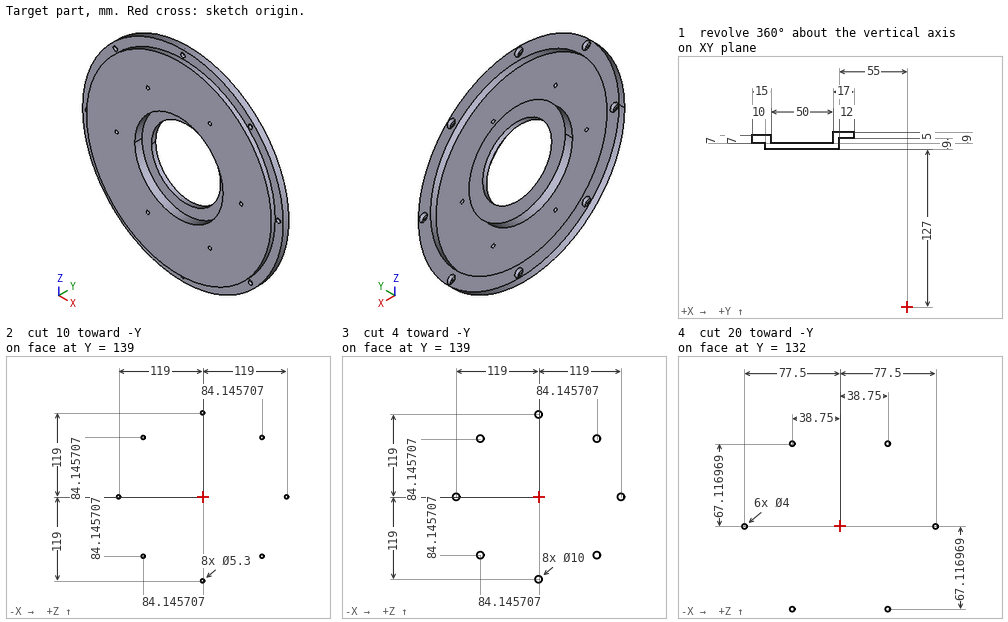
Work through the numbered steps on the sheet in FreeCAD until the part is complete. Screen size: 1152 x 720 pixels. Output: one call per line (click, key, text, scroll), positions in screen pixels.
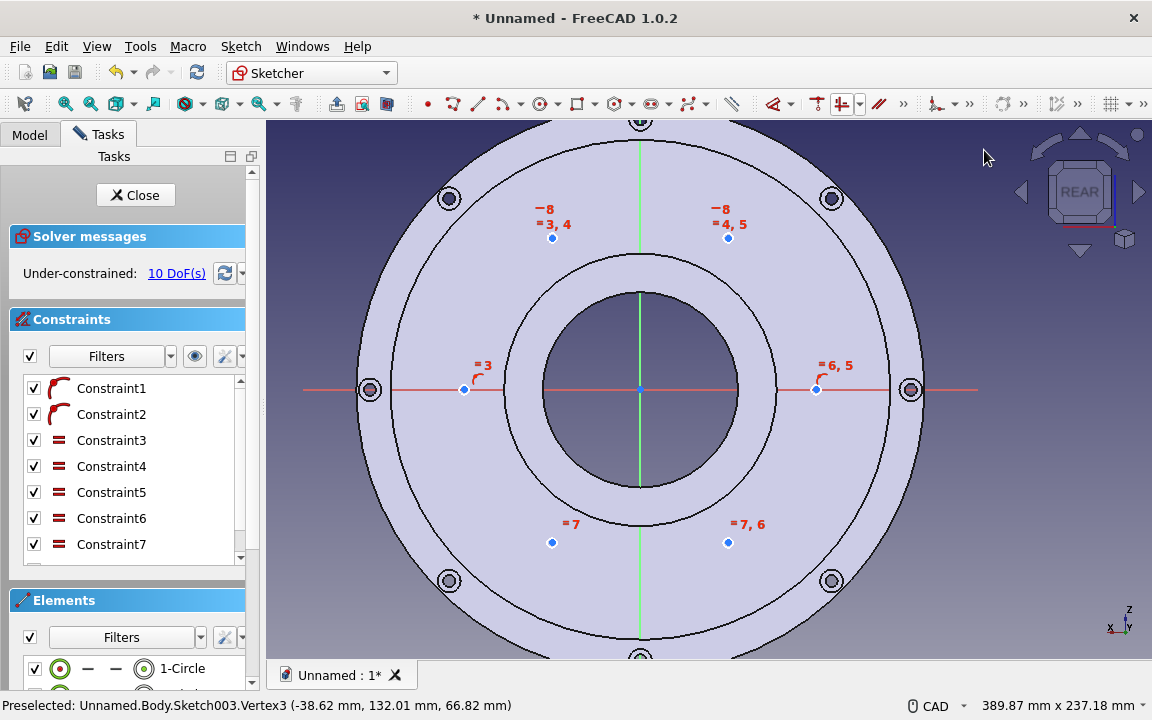
click(728, 238)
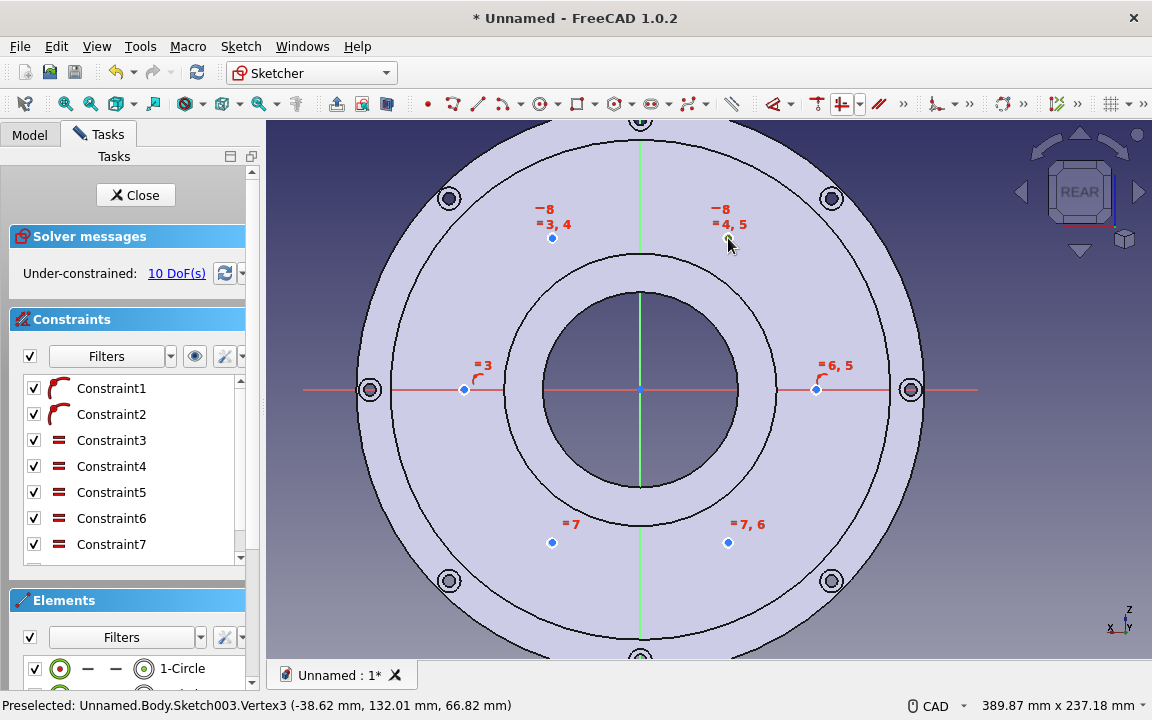
click(728, 543)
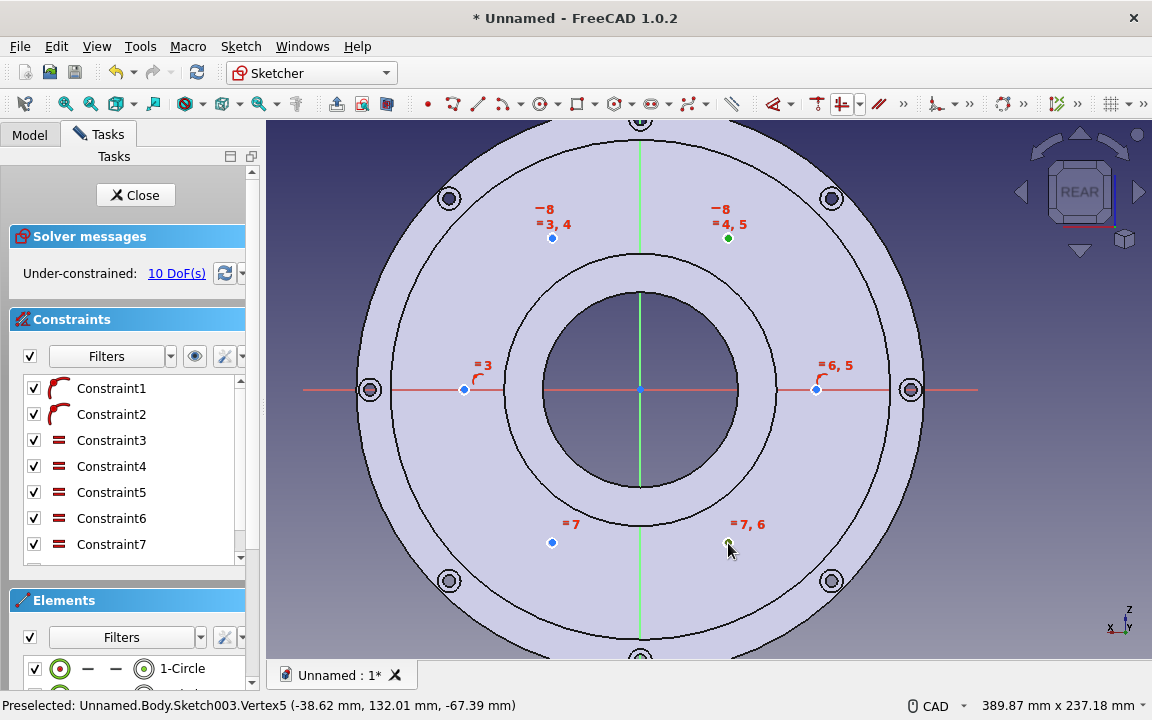
key(v)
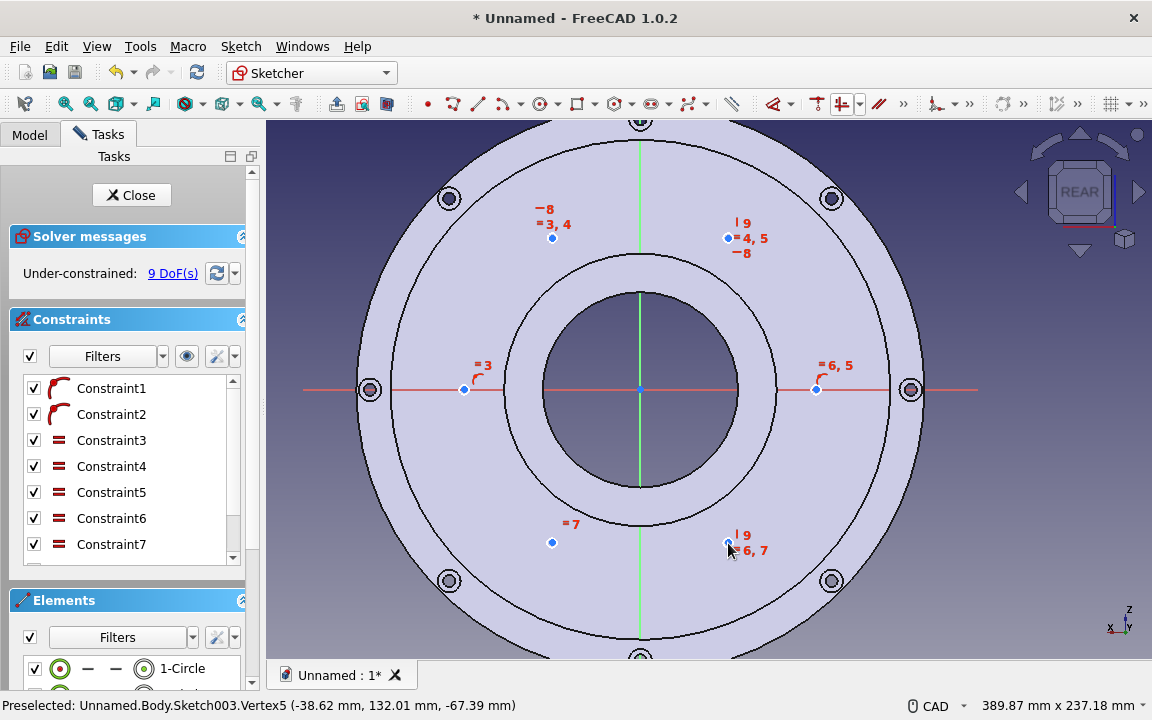
click(552, 238)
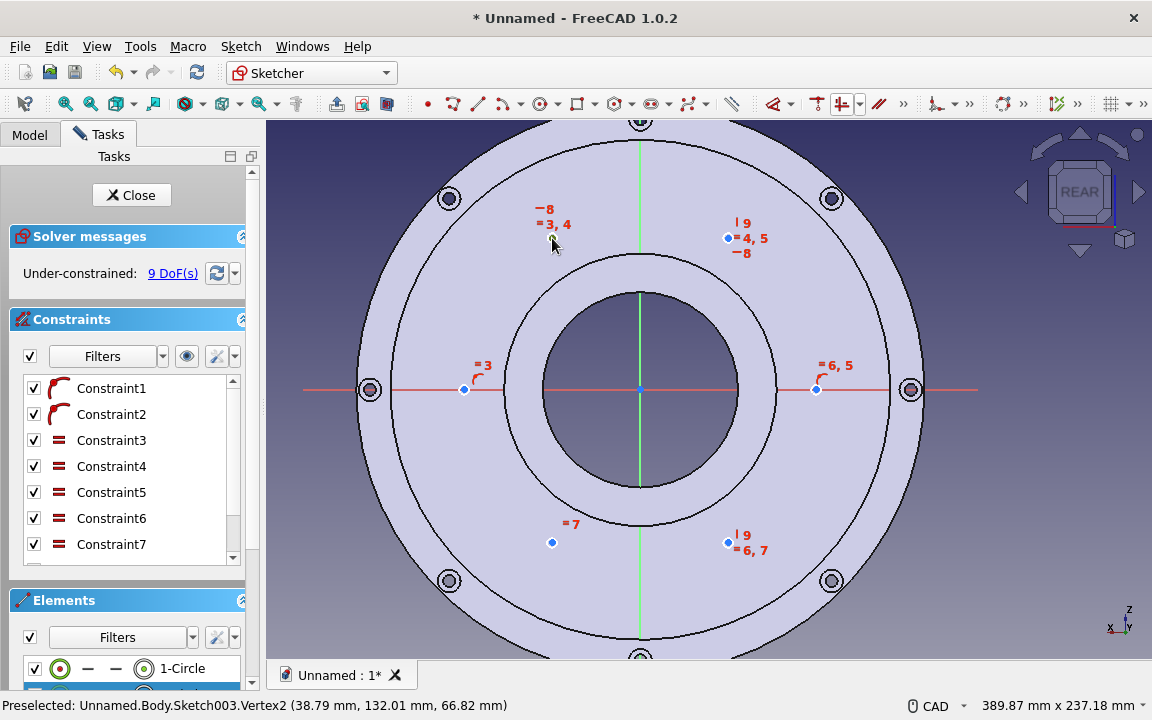
click(552, 543)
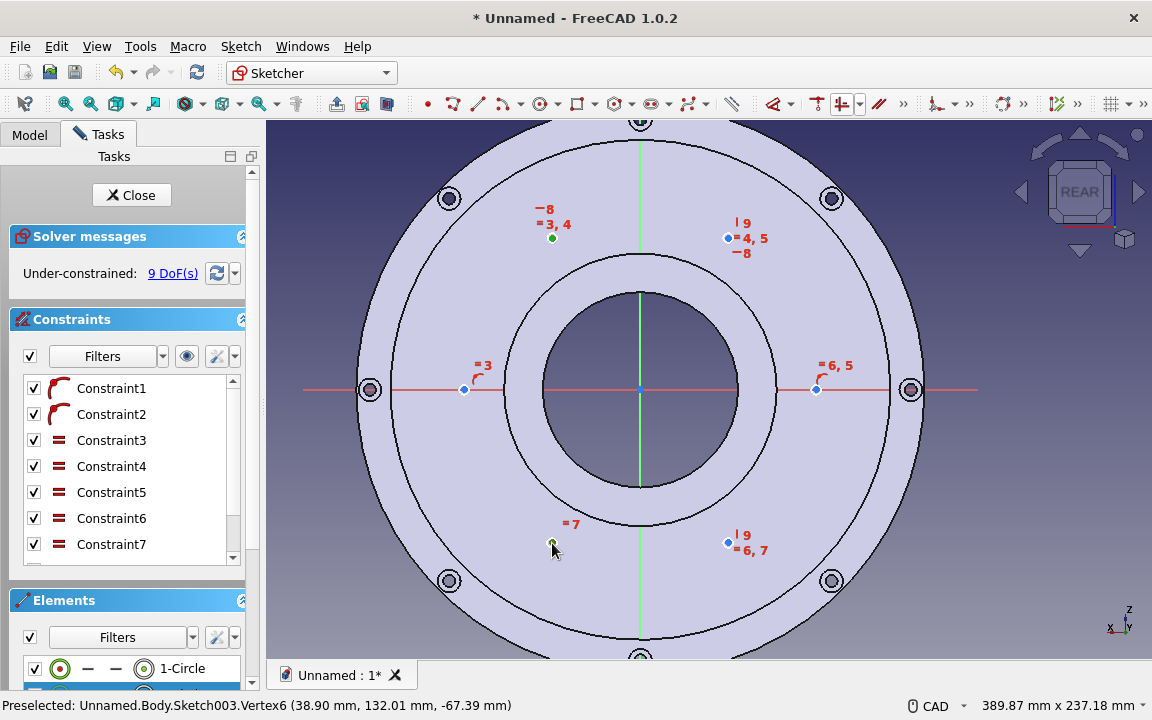
click(860, 104)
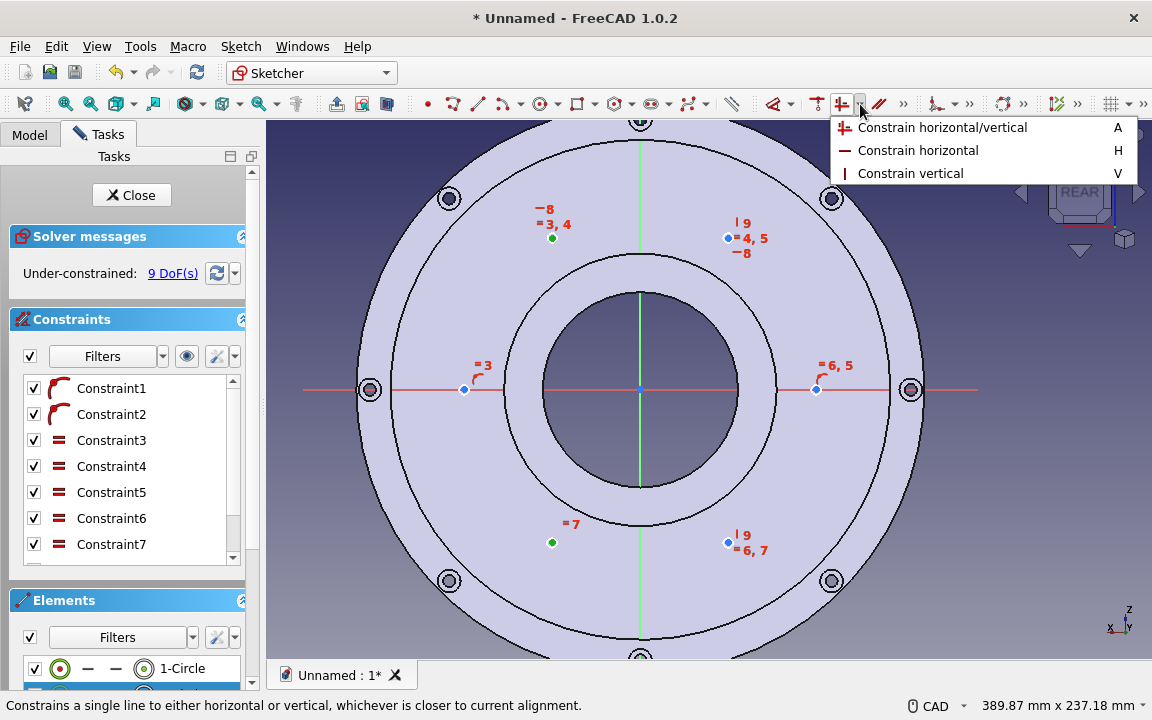
click(984, 174)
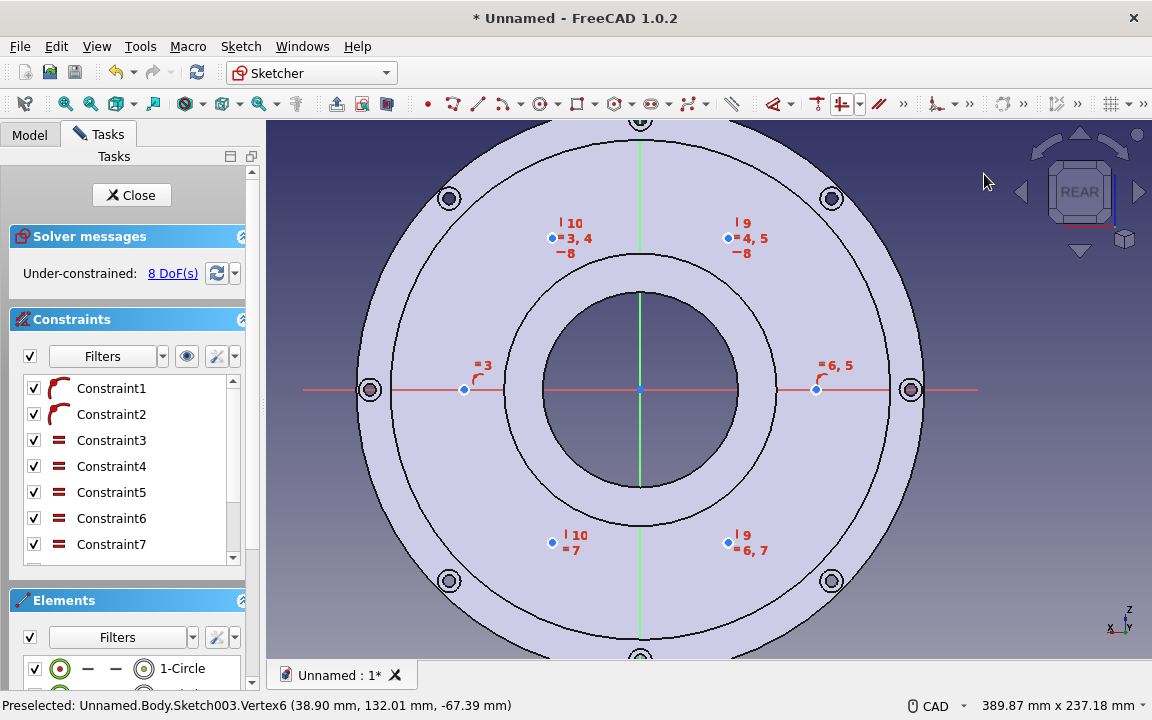
click(728, 543)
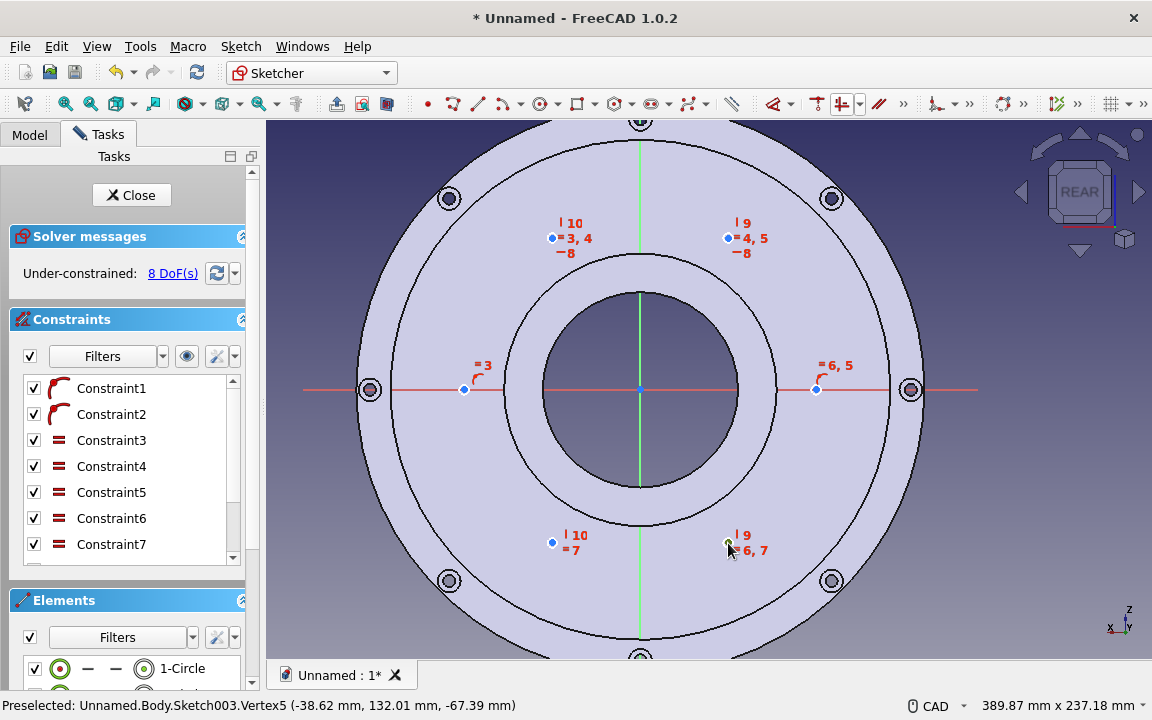
click(552, 543)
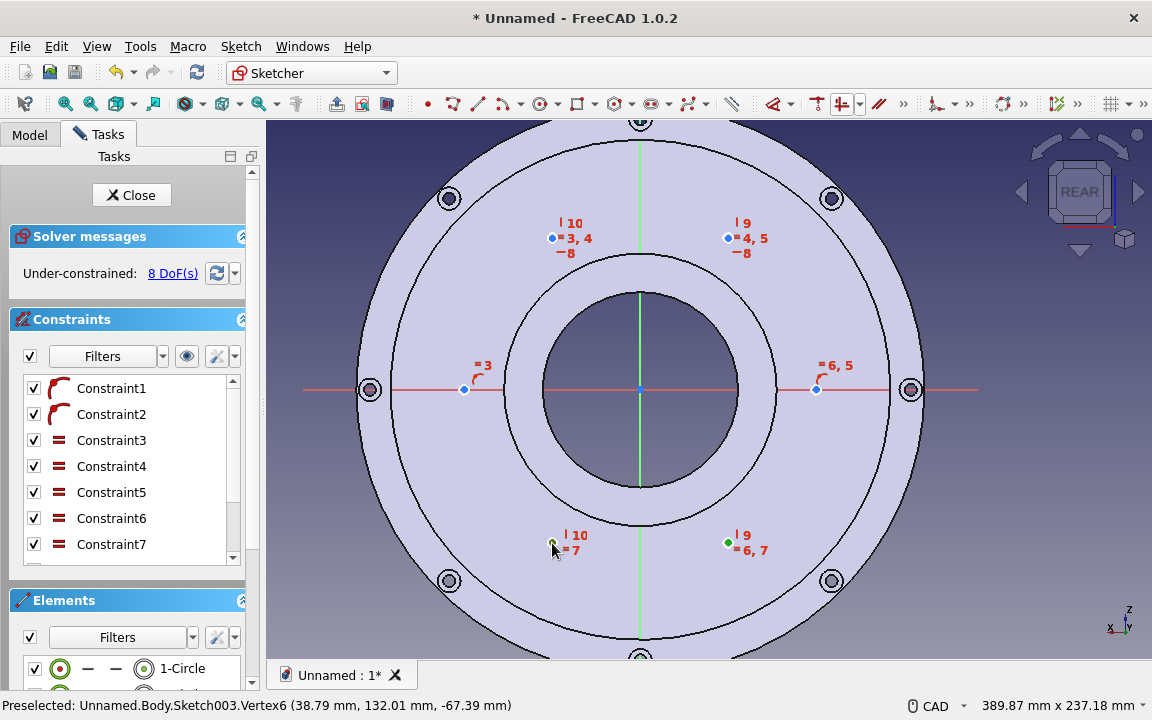
key(h)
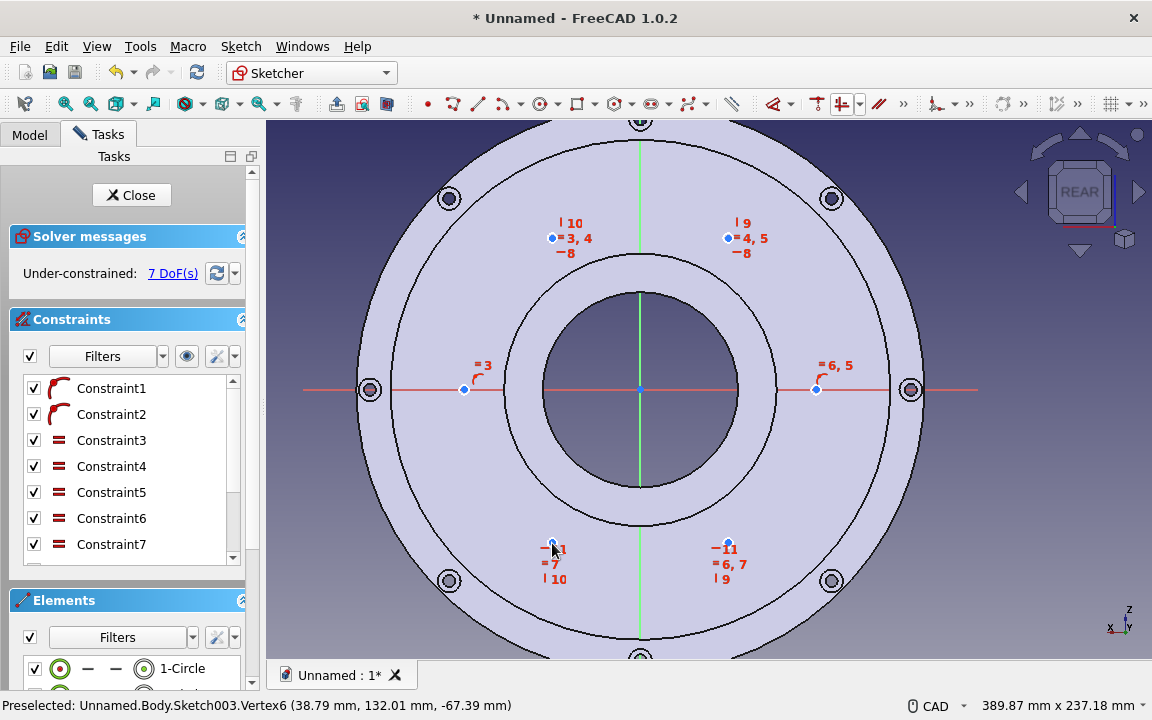
click(772, 104)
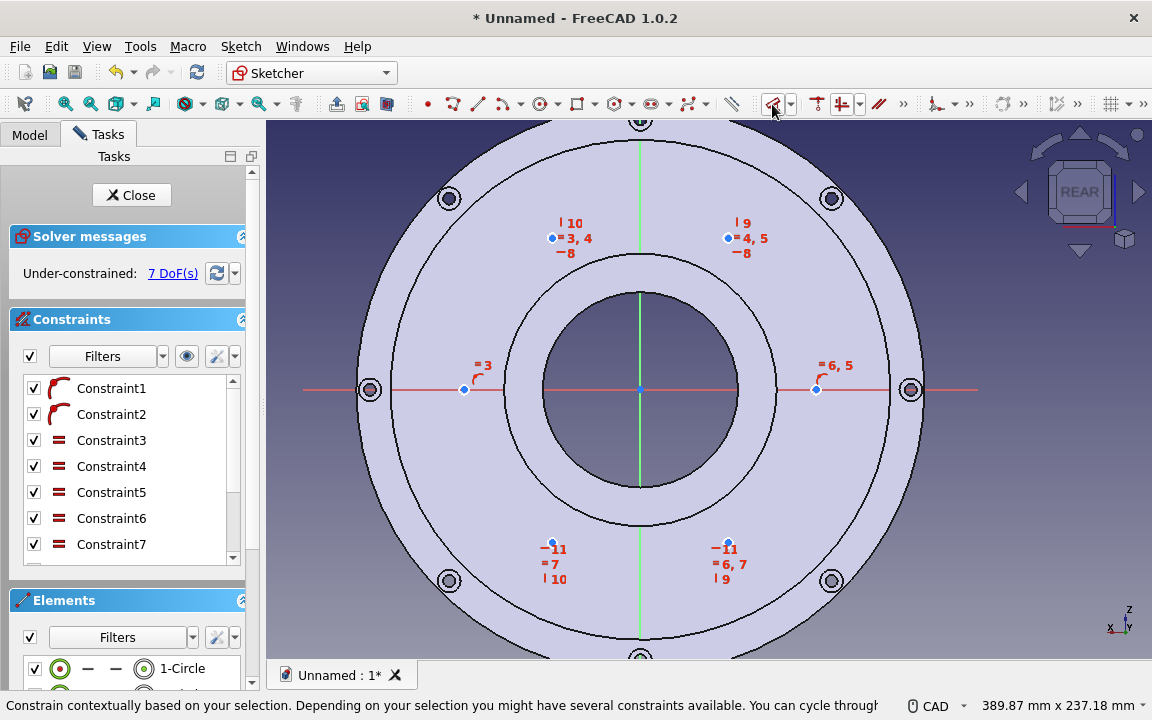
scroll(467, 393, up, 8)